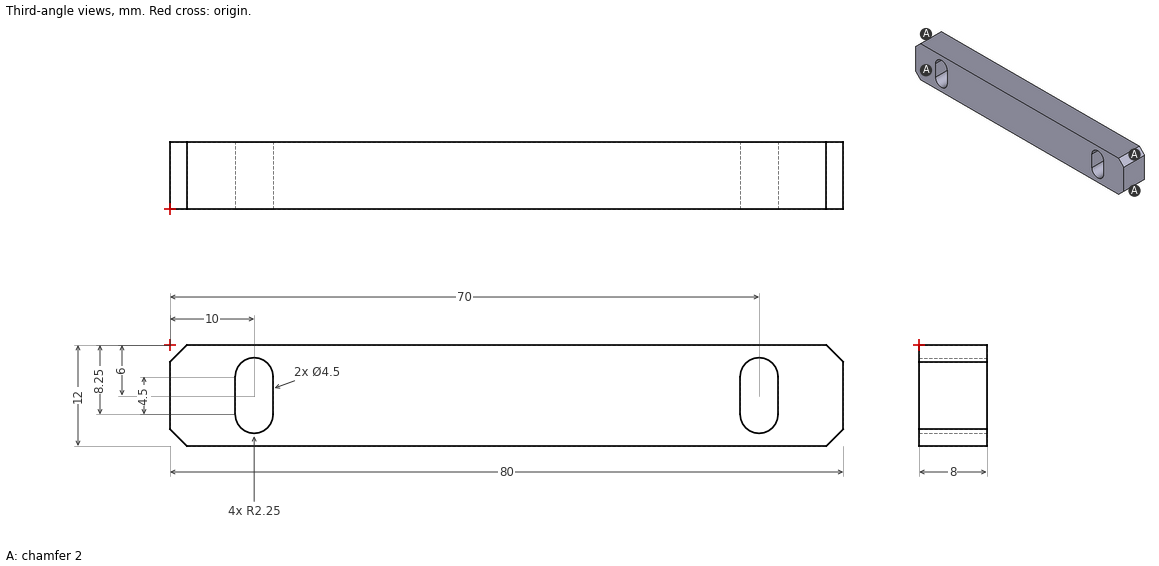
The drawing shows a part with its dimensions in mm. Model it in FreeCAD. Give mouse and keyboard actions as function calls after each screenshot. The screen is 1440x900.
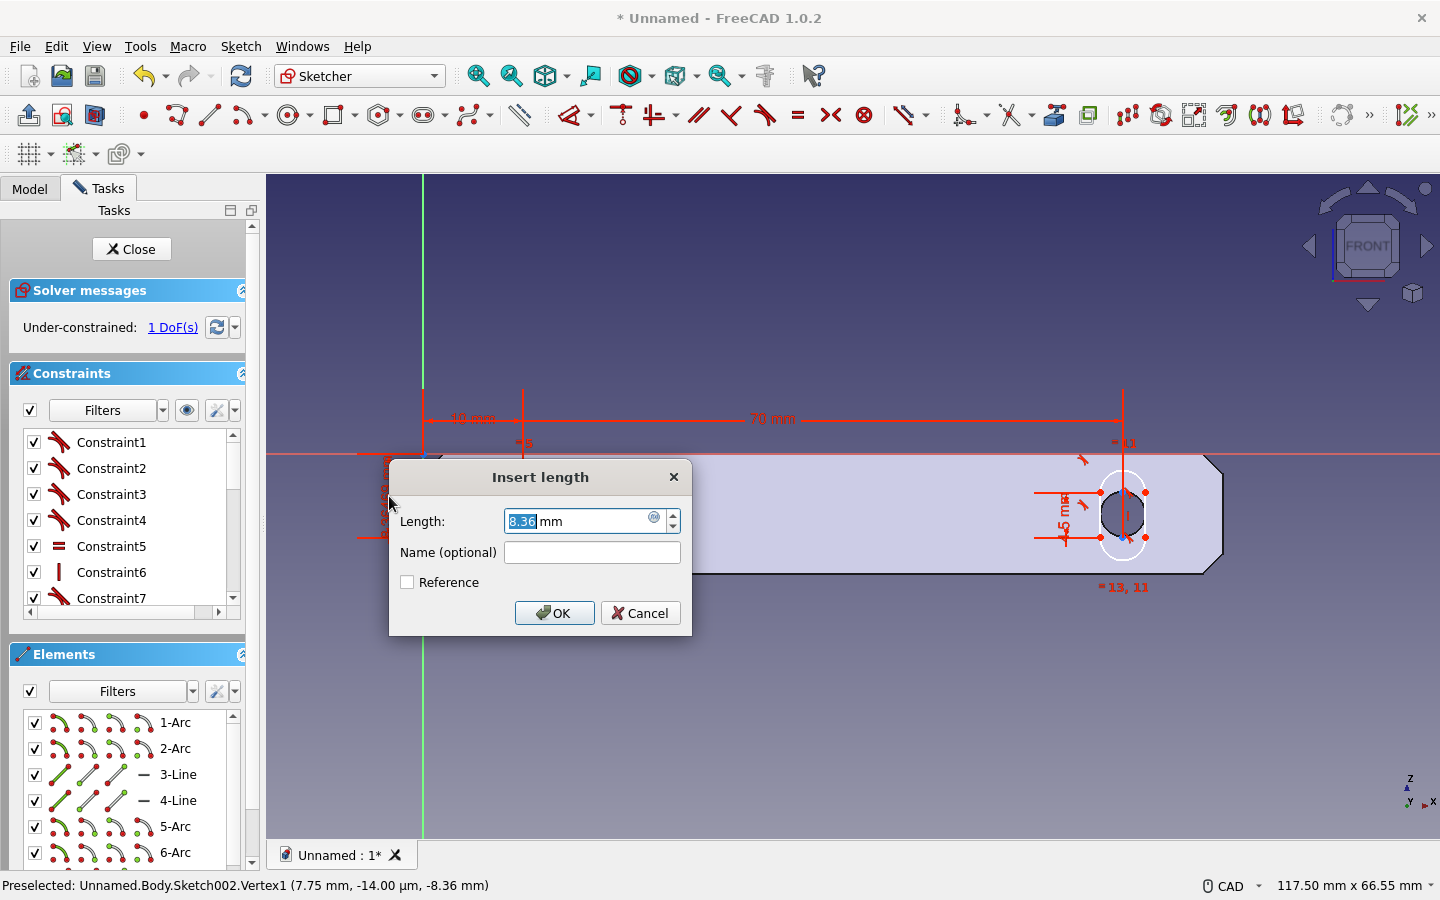
text(8.25)
key(Return)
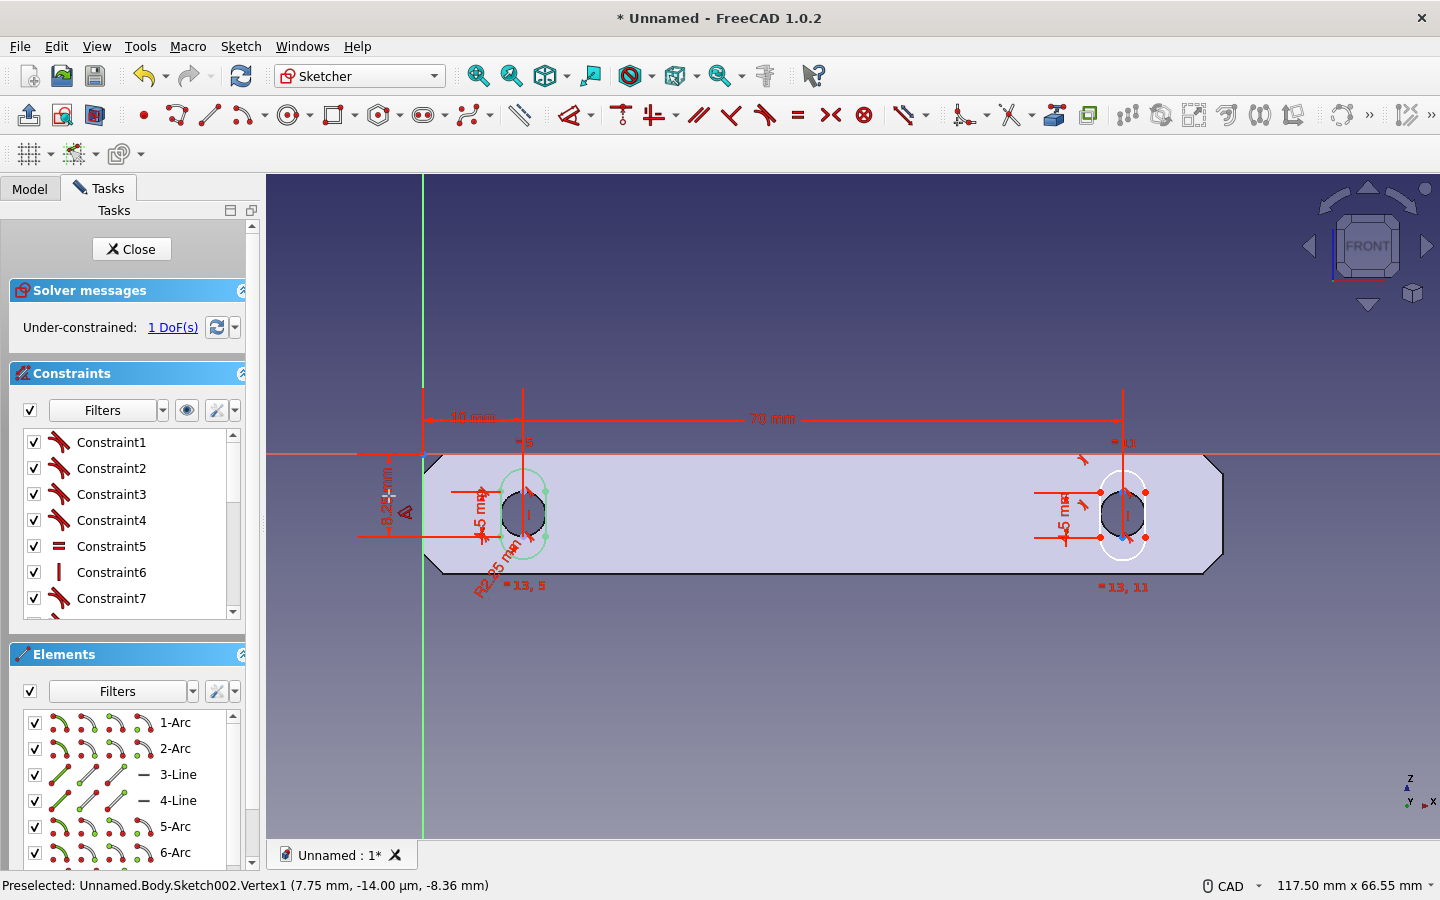
click(1100, 538)
click(389, 525)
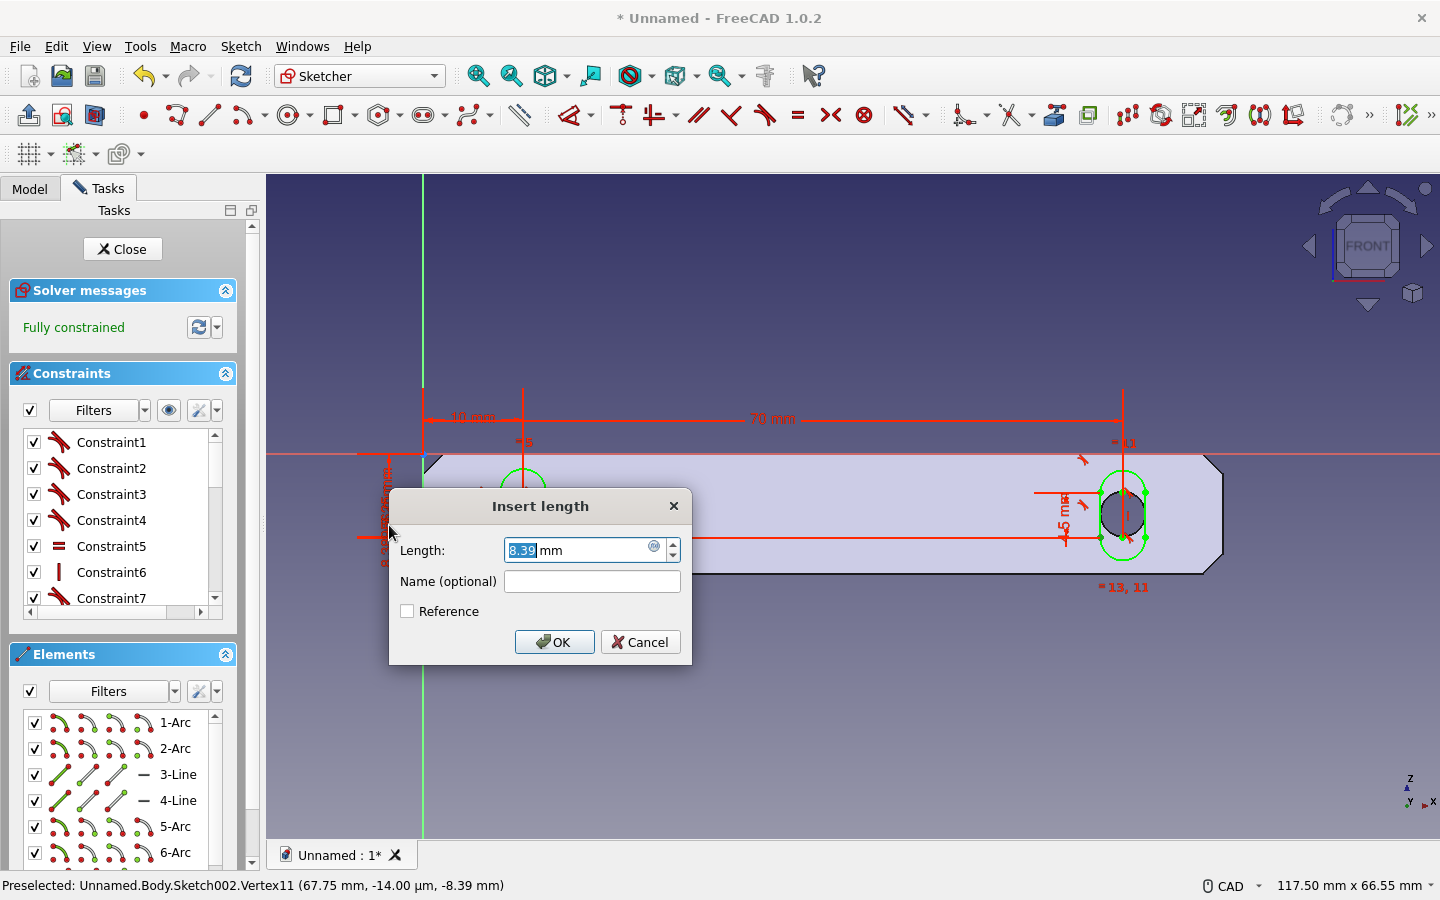
text(8.25)
key(Return)
key(Escape)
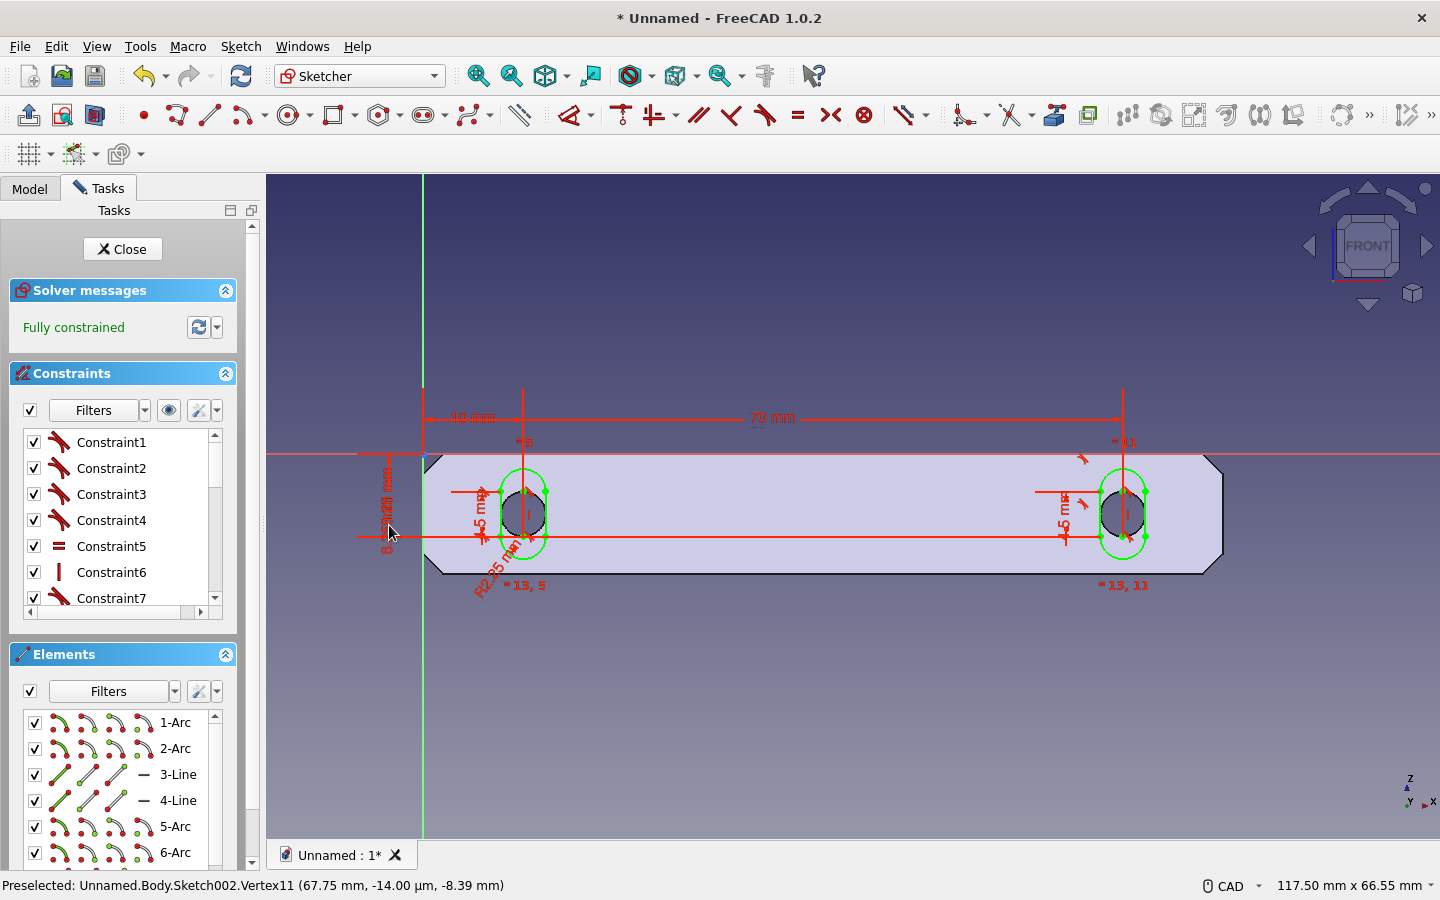
click(123, 249)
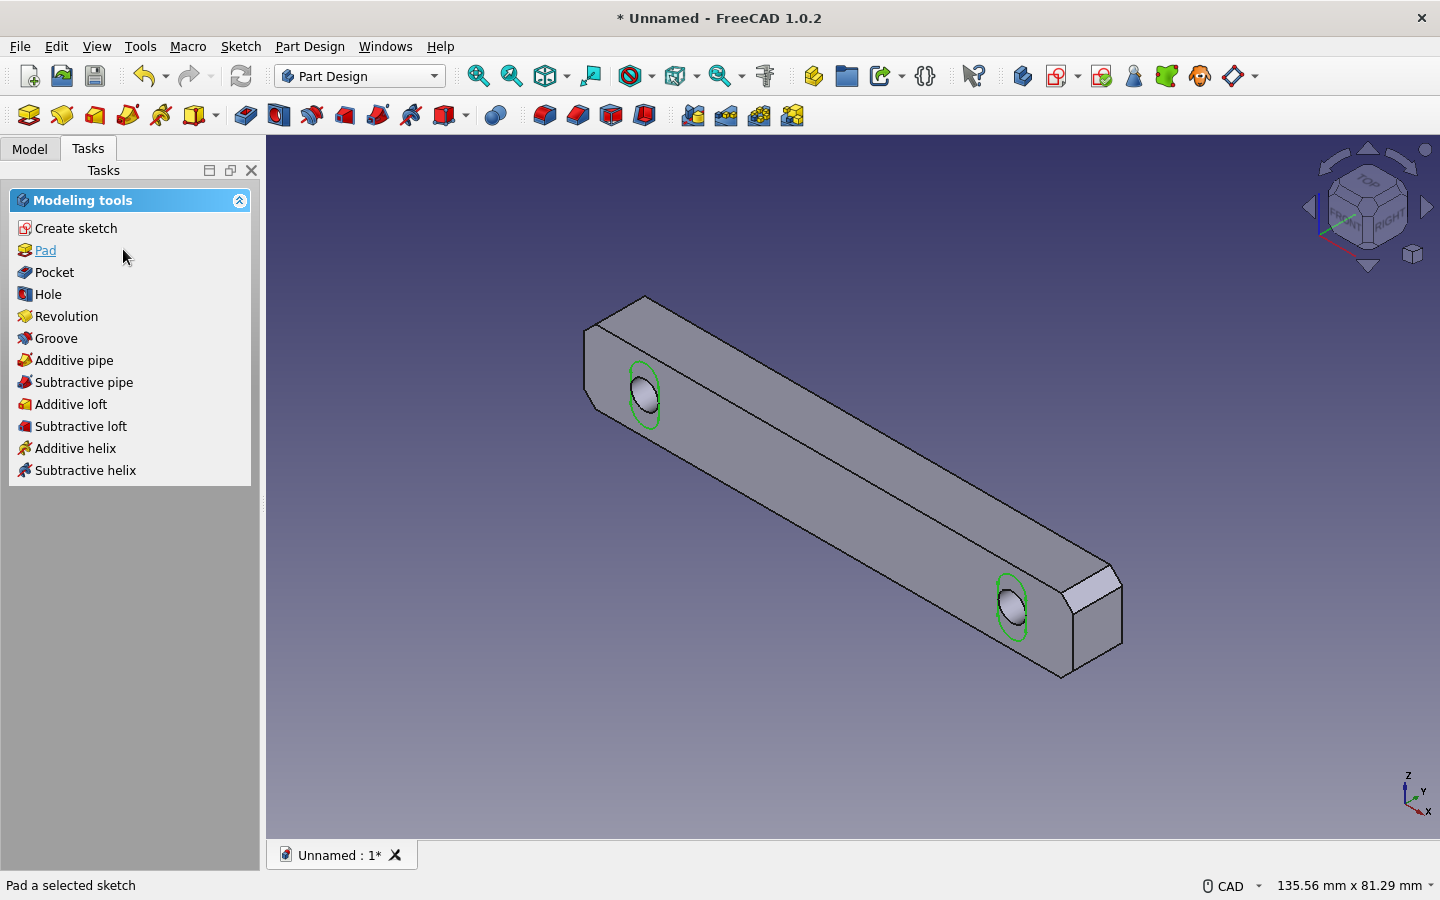
click(246, 116)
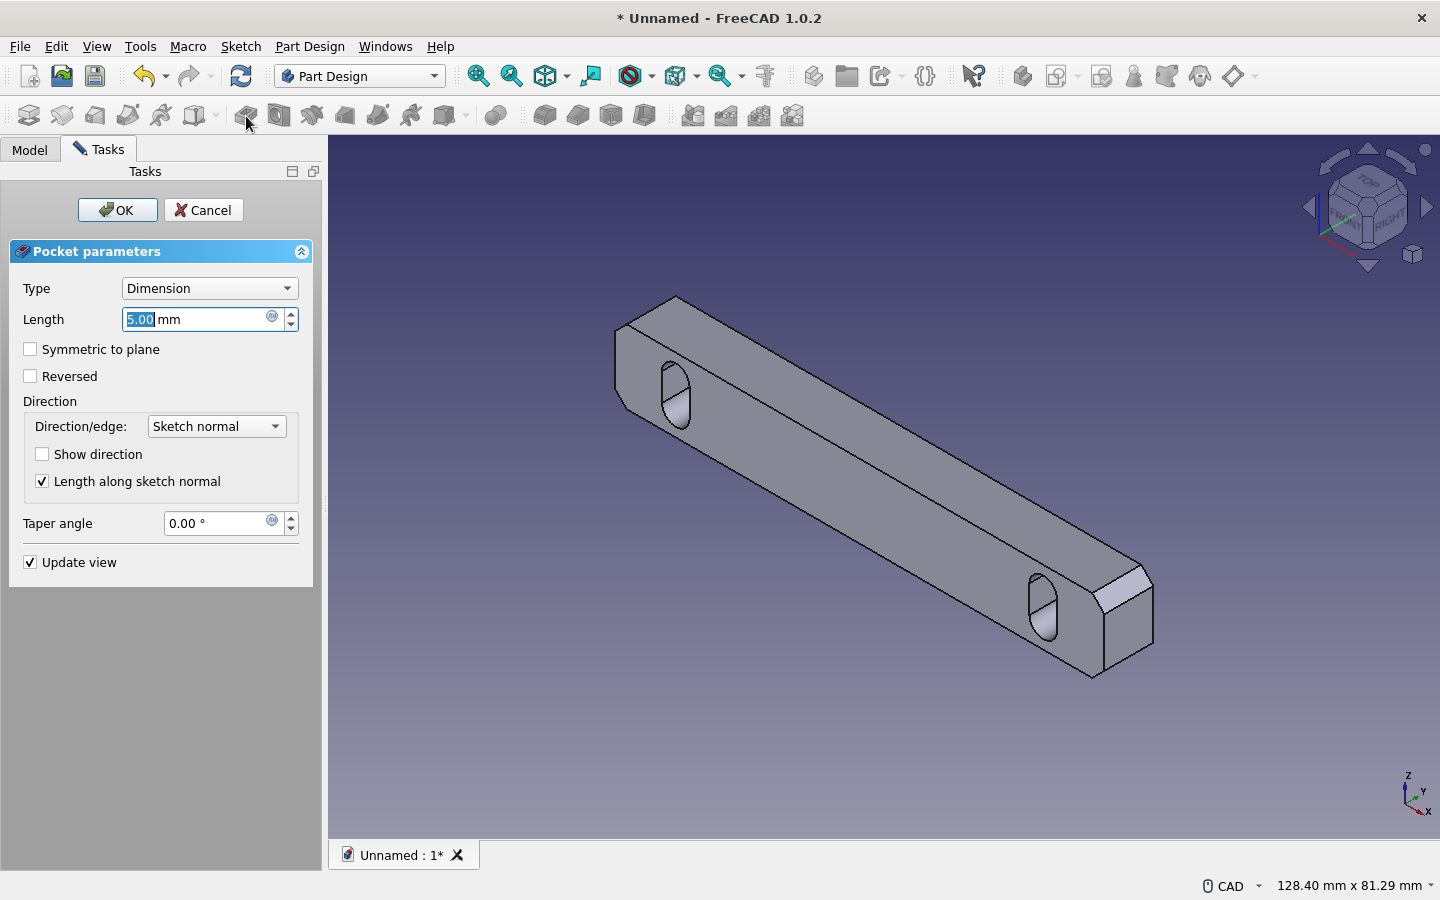
text(10)
key(Tab)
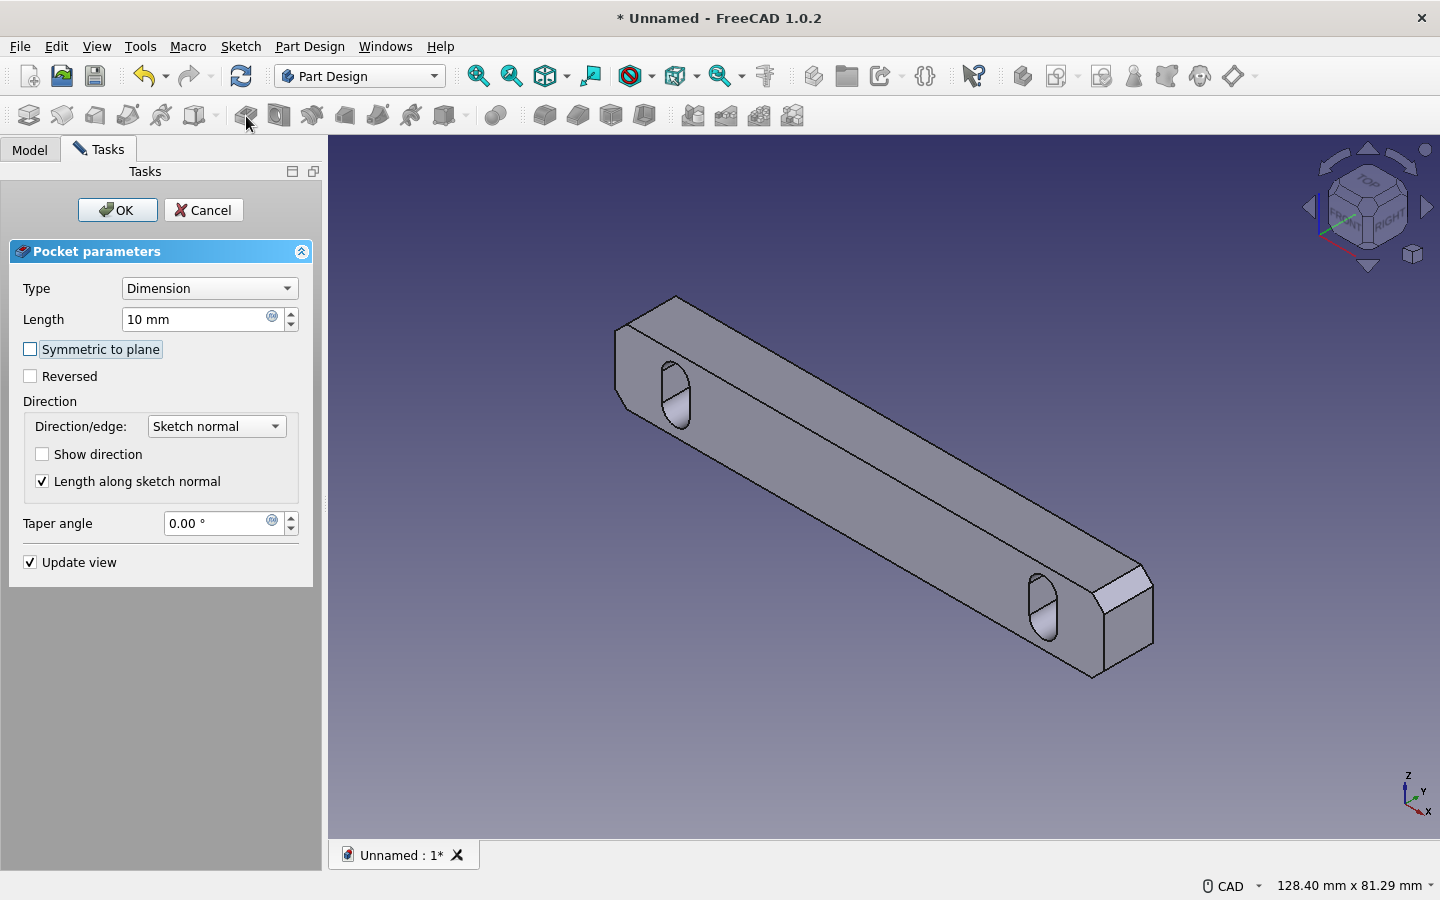
click(118, 210)